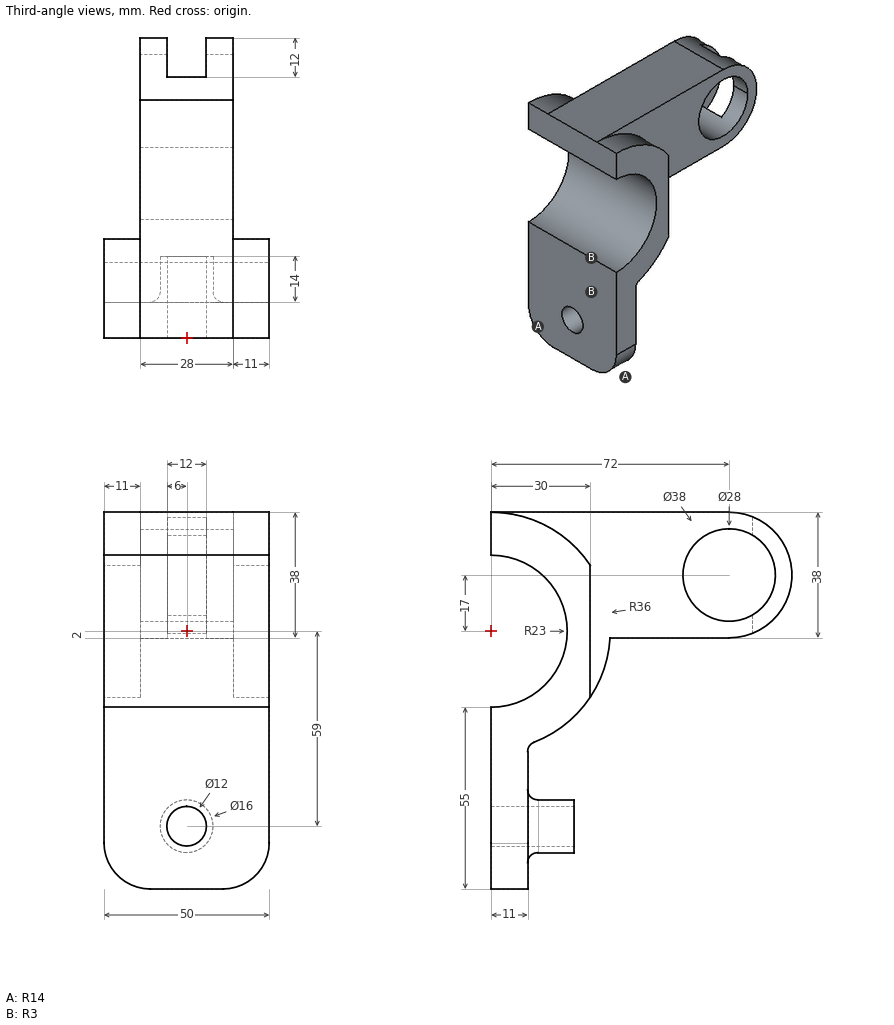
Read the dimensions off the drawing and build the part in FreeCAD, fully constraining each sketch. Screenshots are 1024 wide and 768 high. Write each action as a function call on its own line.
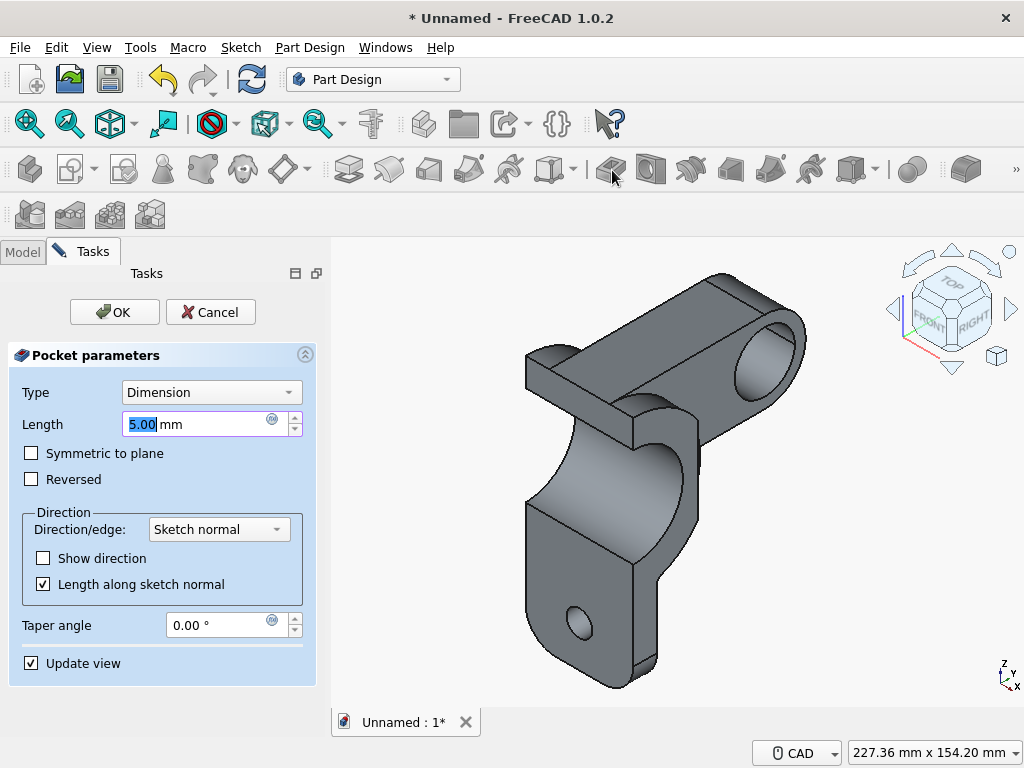
text(11)
key(Tab)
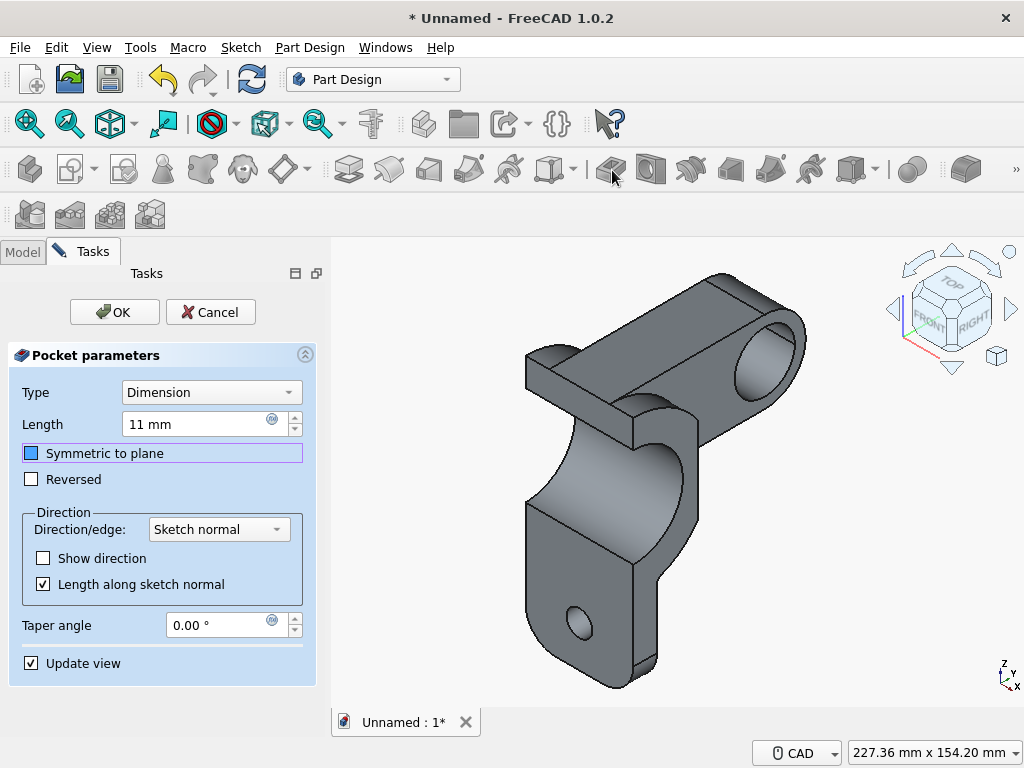
click(115, 312)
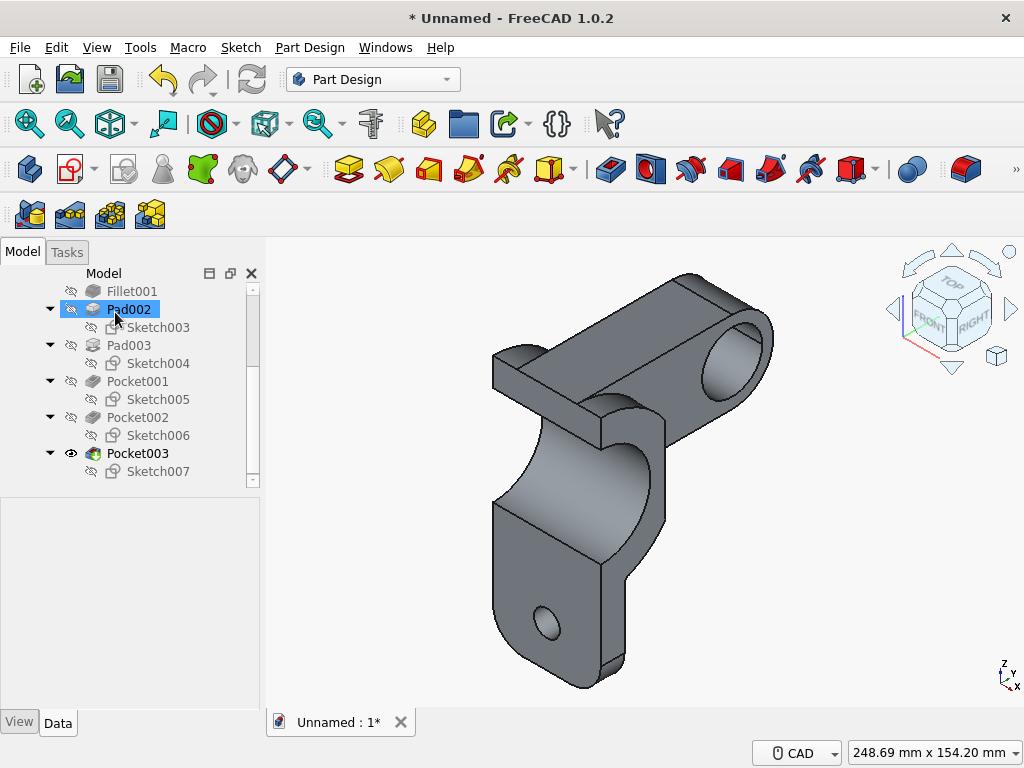
scroll(140, 377, down, 3)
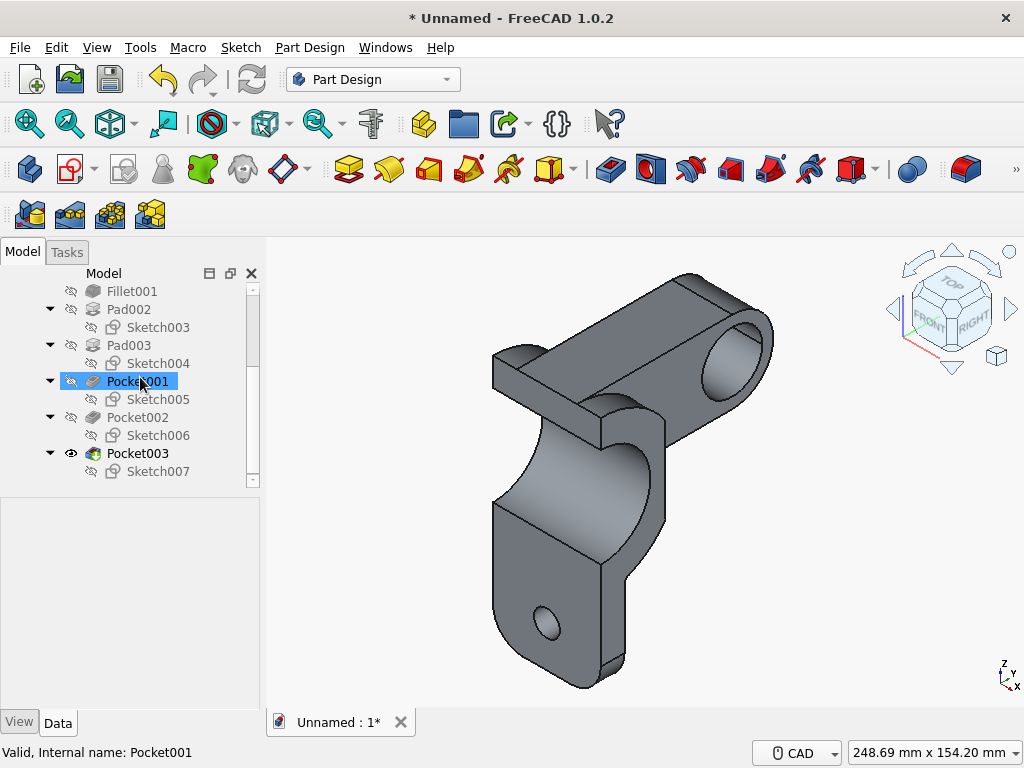
scroll(140, 377, up, 15)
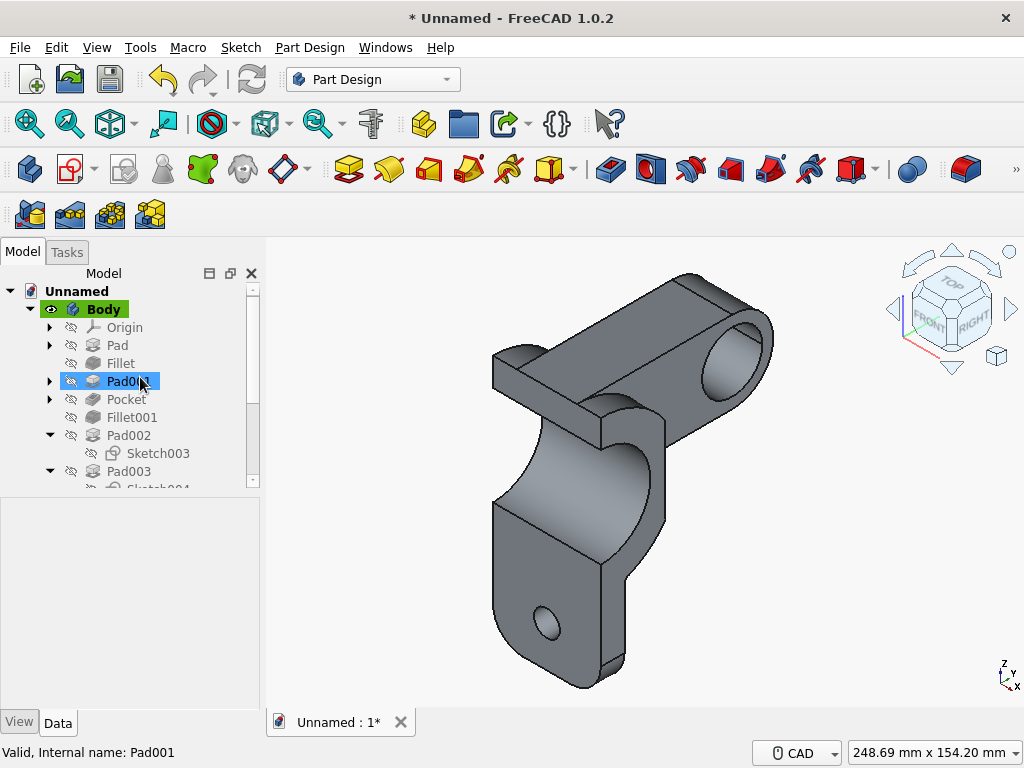
click(50, 327)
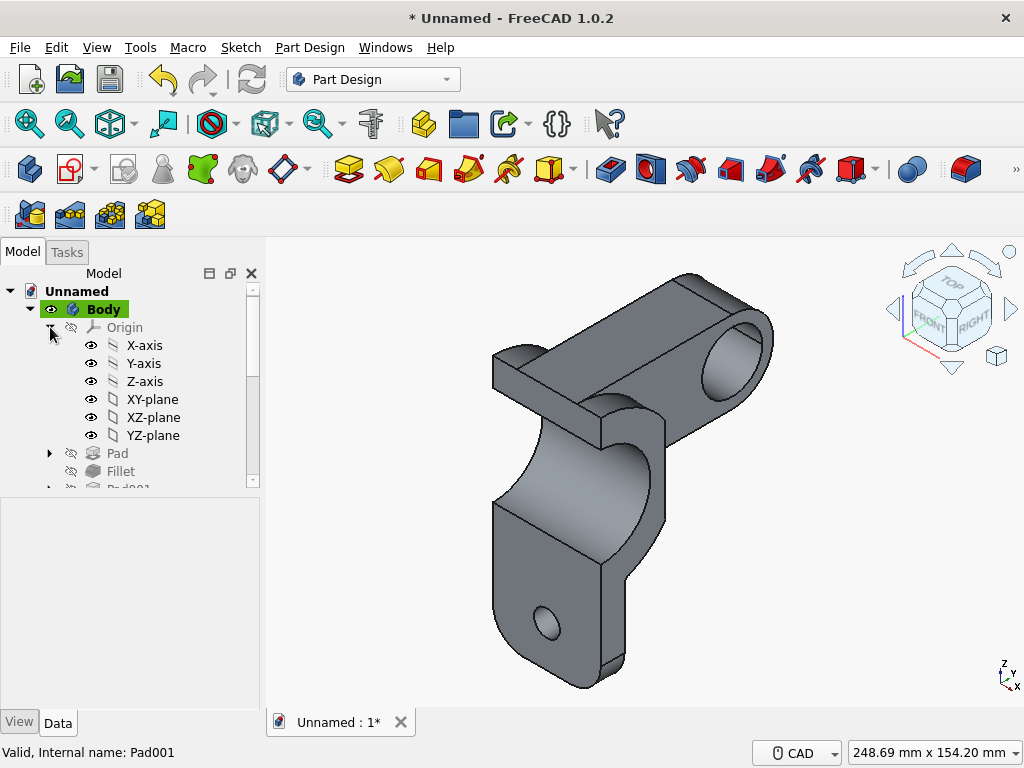
click(136, 417)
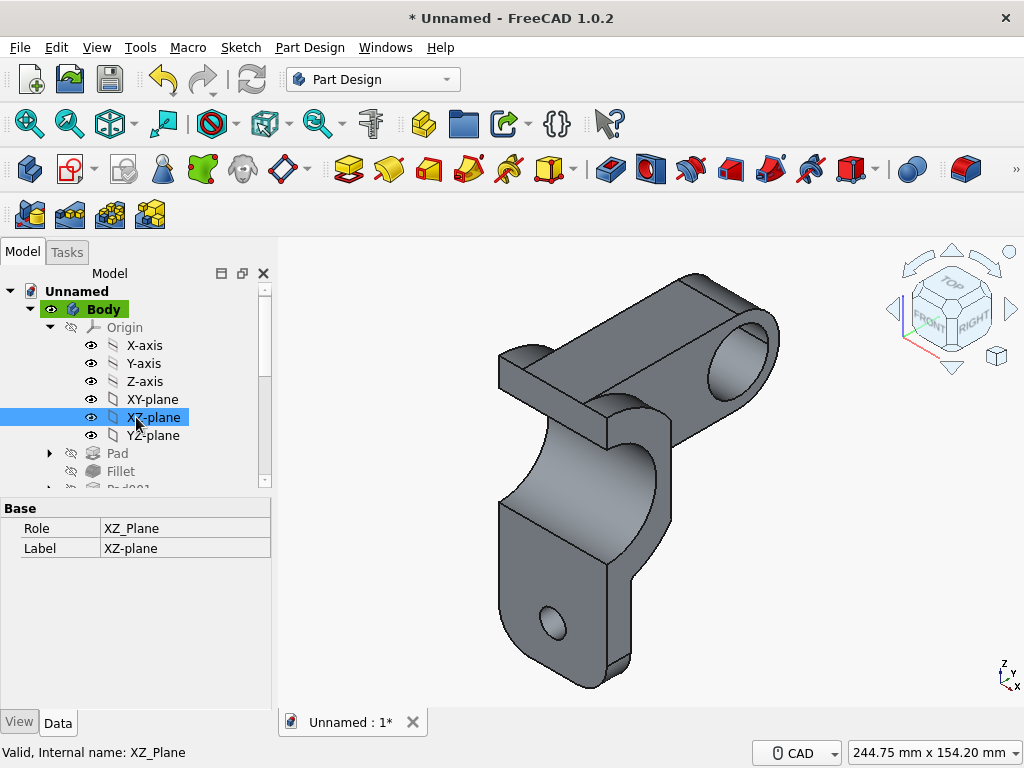
click(284, 170)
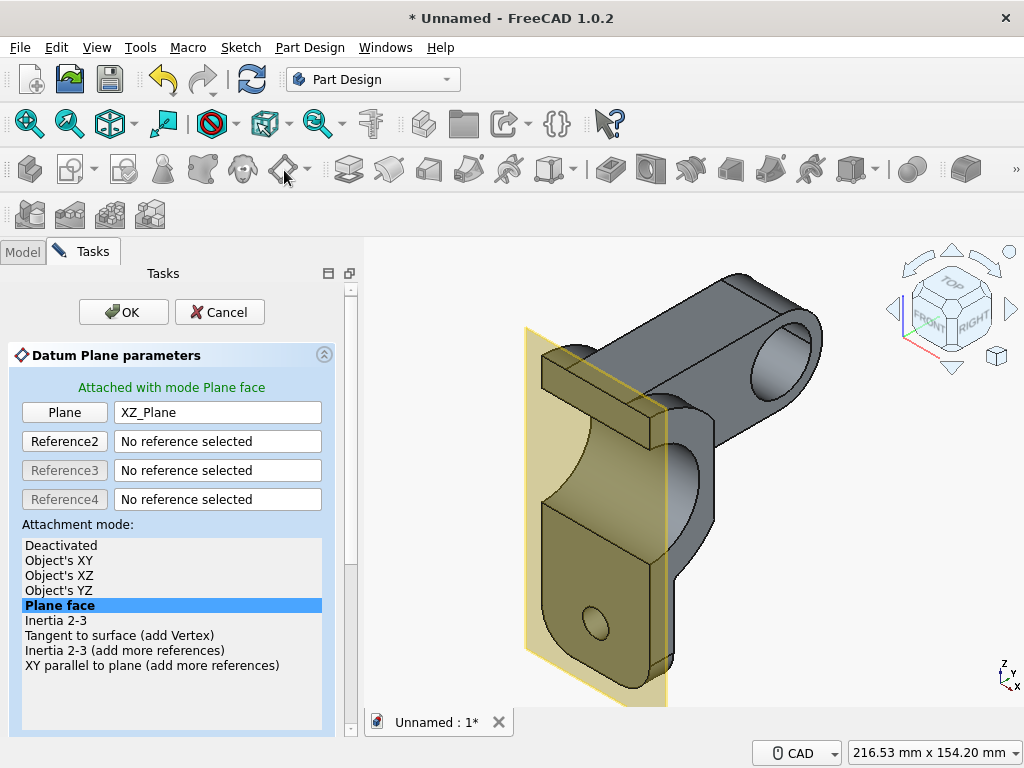
scroll(351, 510, down, 3)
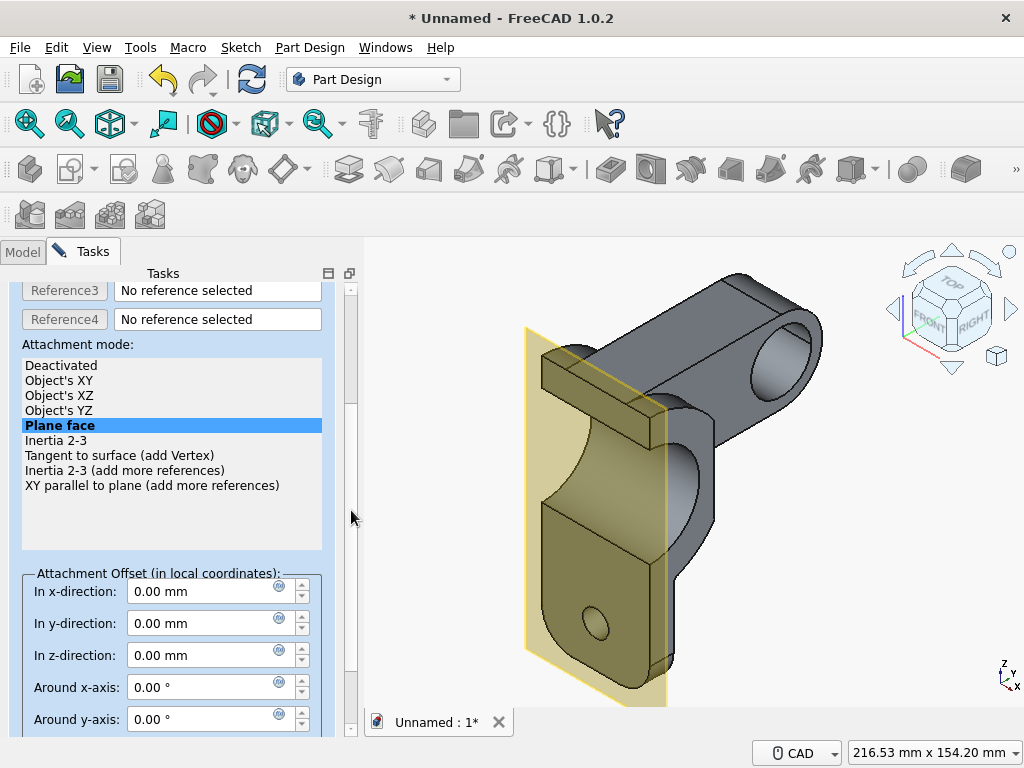
triple_click(210, 655)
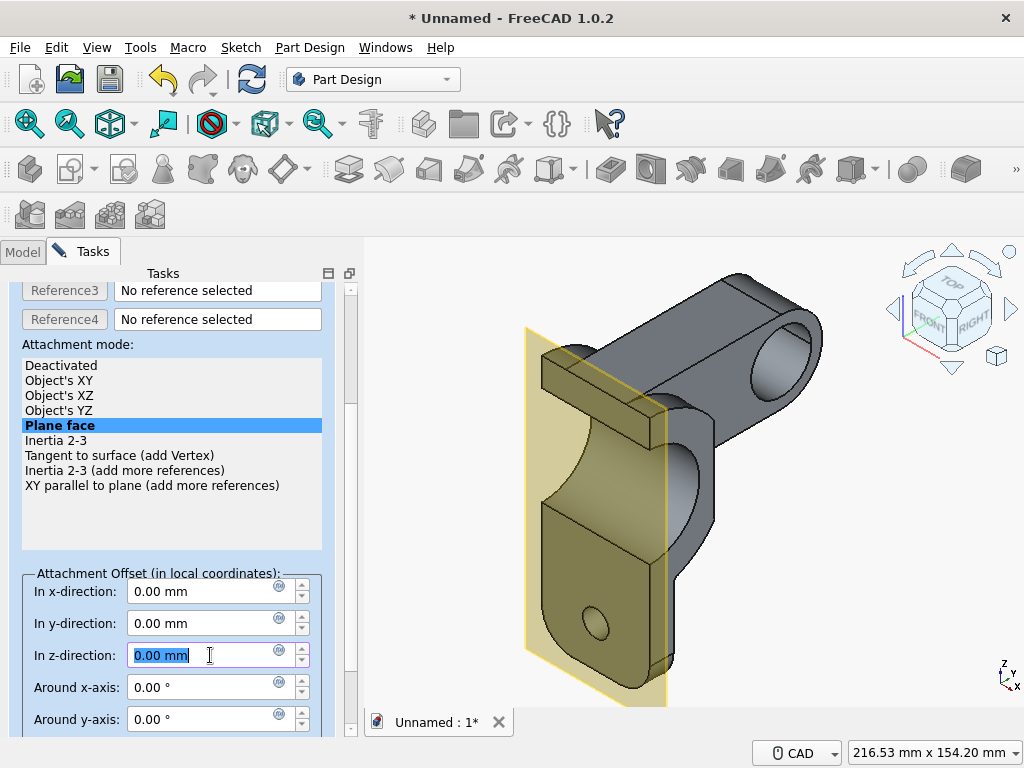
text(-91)
key(Tab)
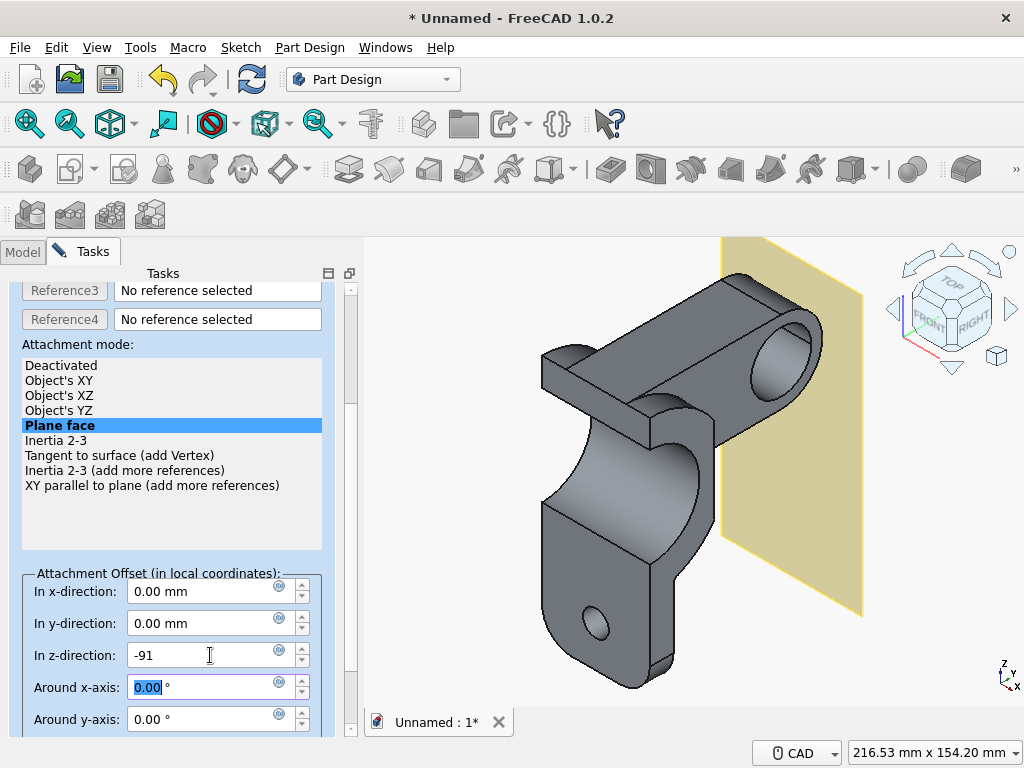
scroll(351, 510, up, 4)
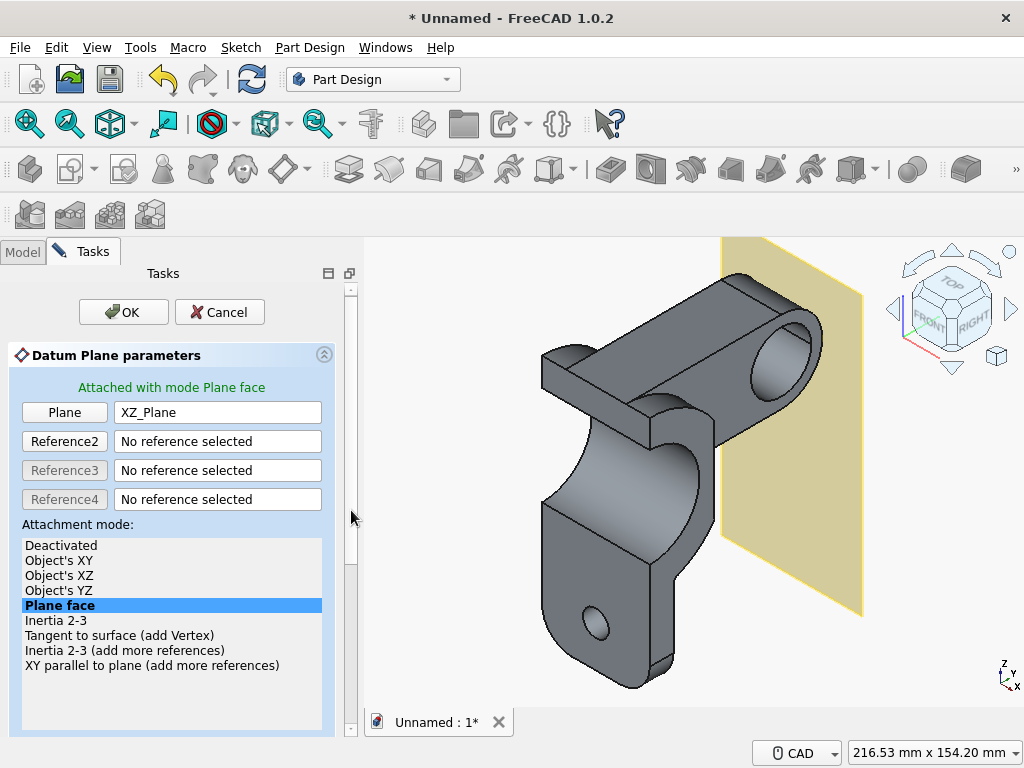
click(124, 312)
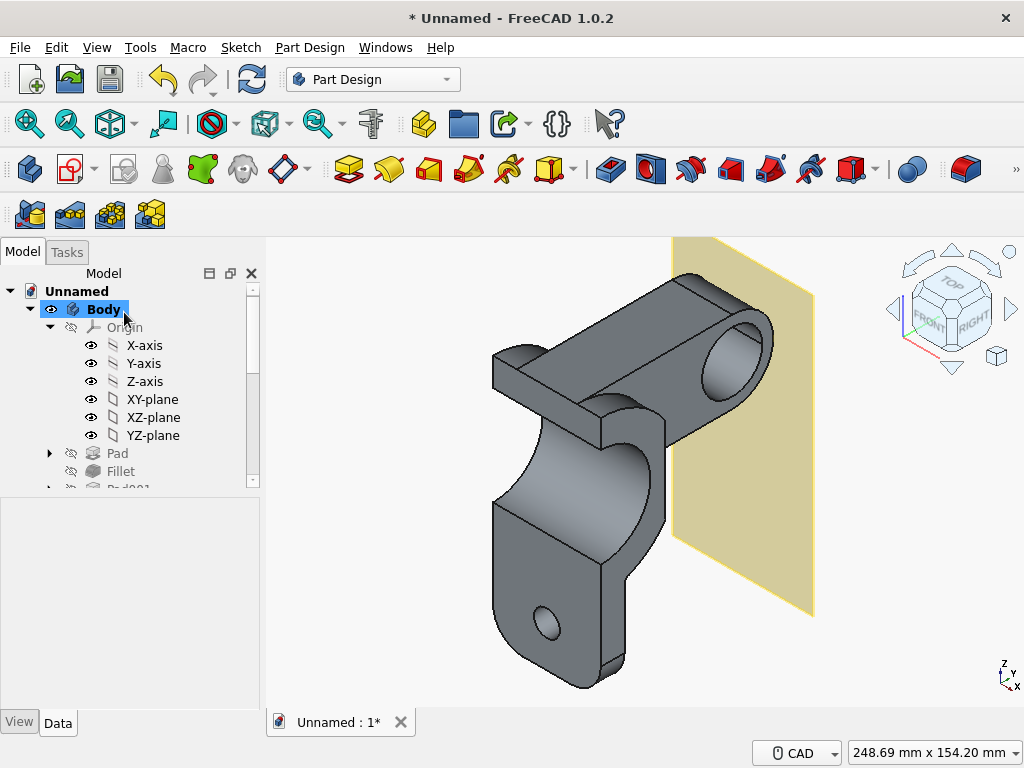
scroll(100, 377, down, 3)